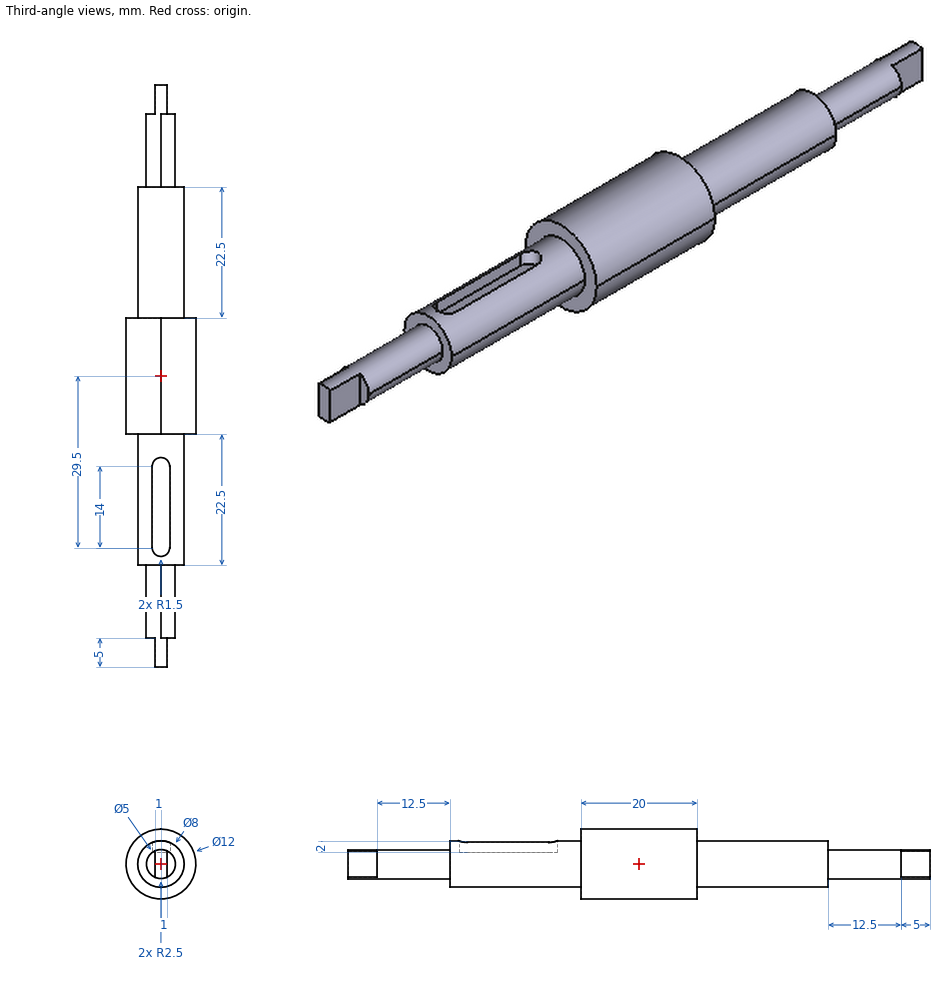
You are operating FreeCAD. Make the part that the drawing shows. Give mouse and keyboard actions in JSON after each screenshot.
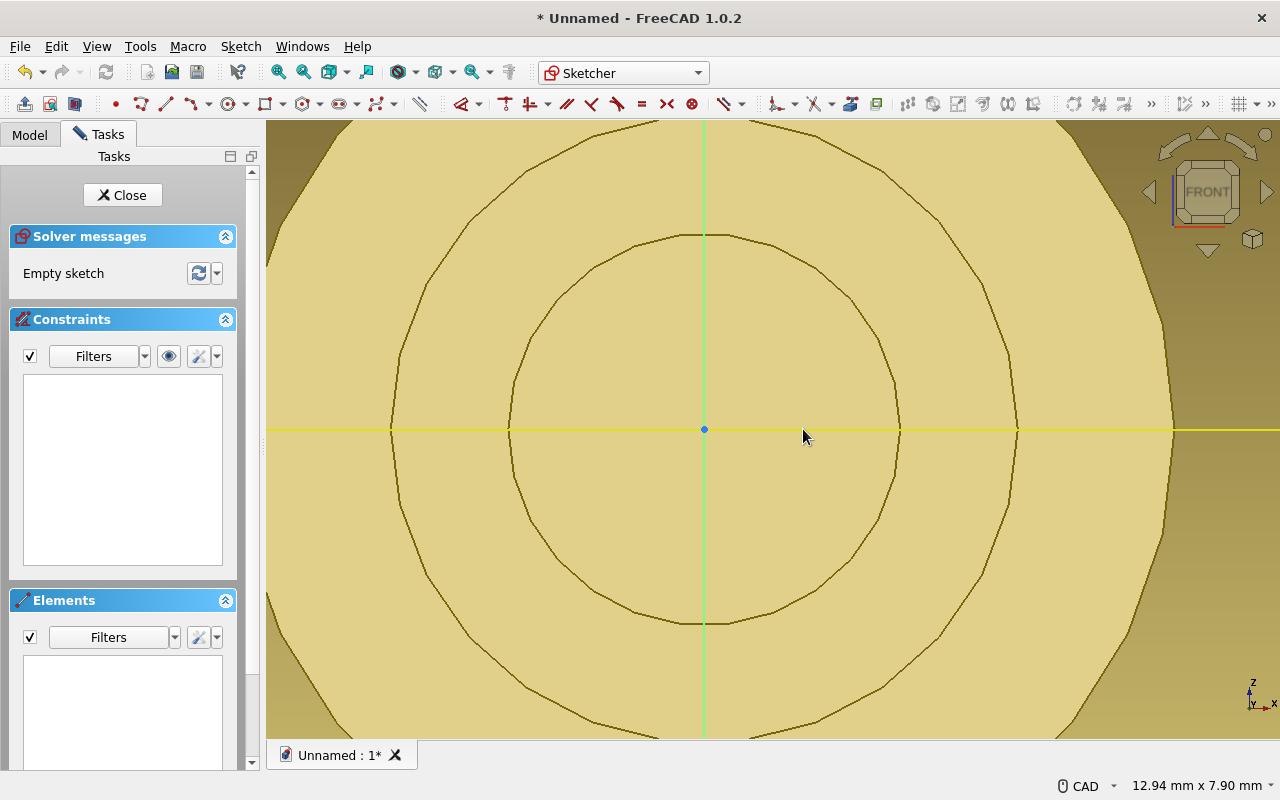
{"action": "left_click", "coordinate": [166, 104]}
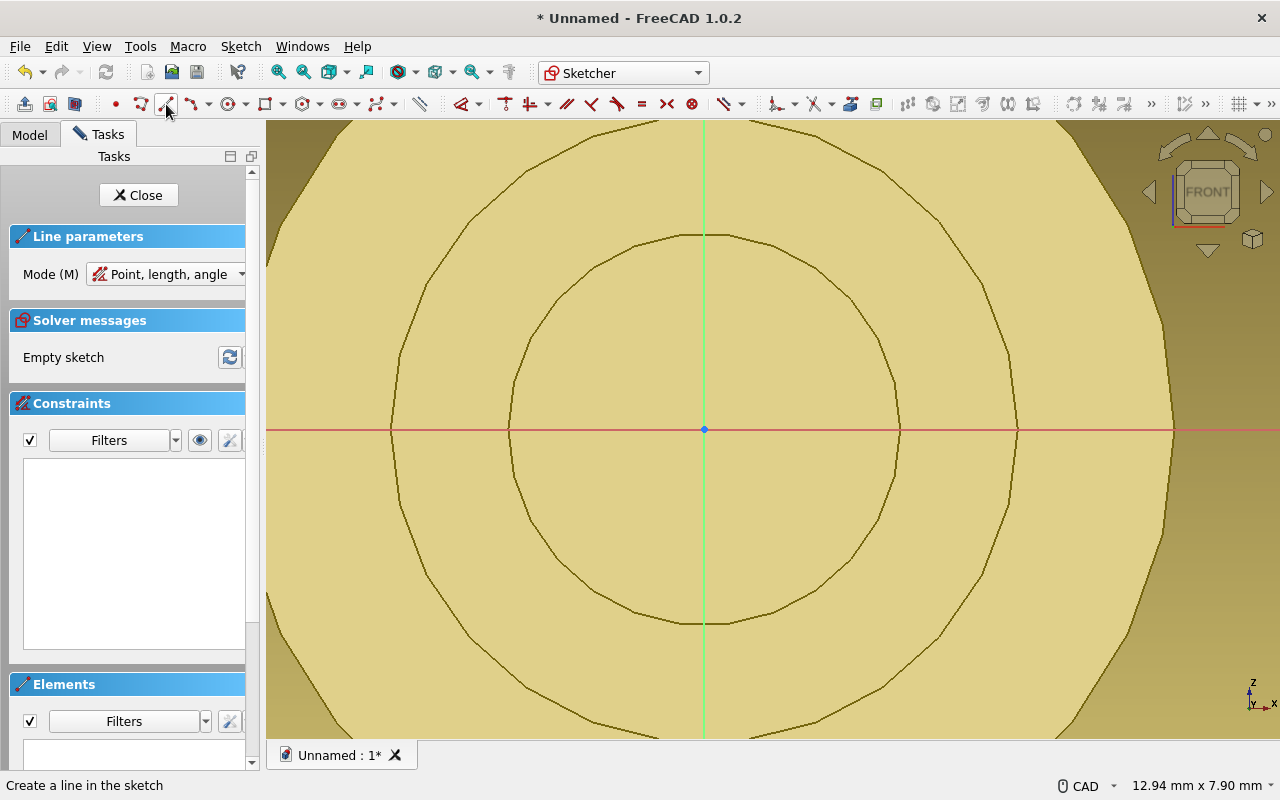
{"action": "left_click", "coordinate": [626, 250]}
{"action": "left_click", "coordinate": [626, 609]}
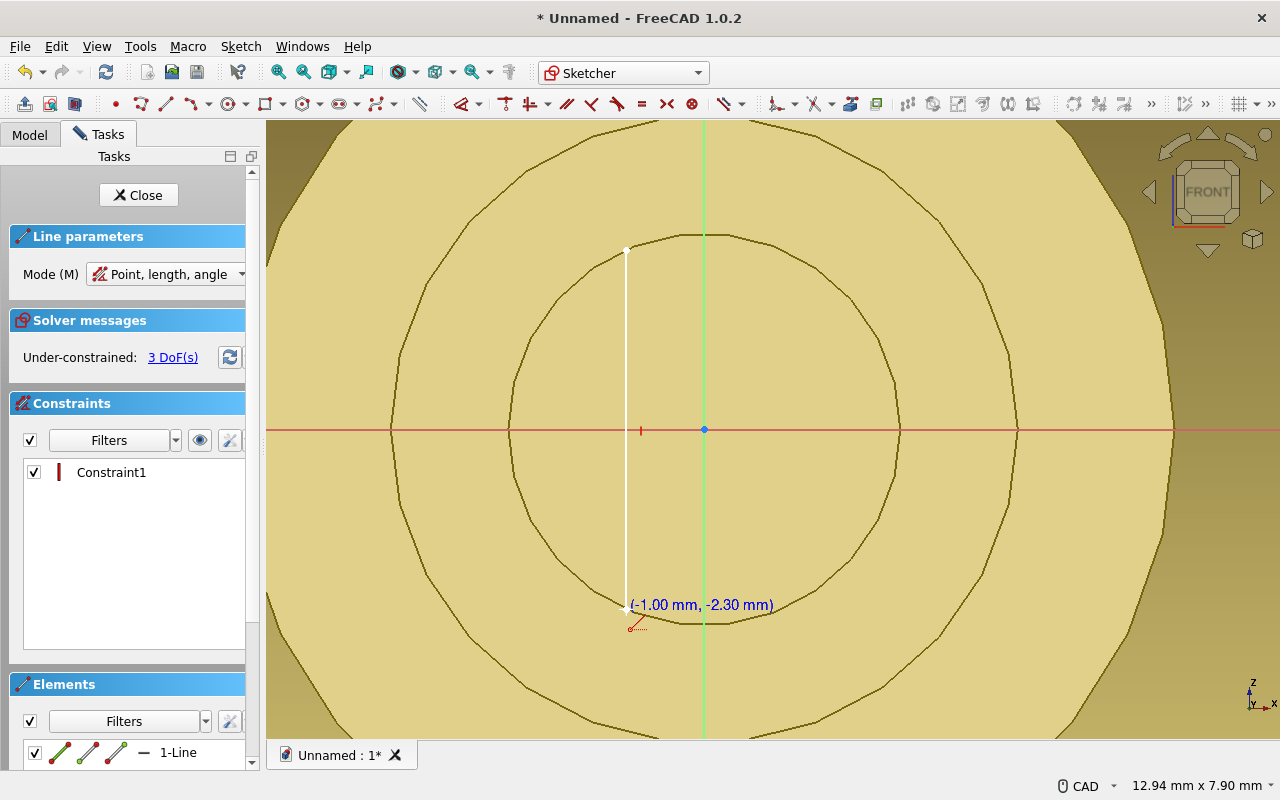
{"action": "left_click", "coordinate": [783, 609]}
{"action": "left_click", "coordinate": [783, 250]}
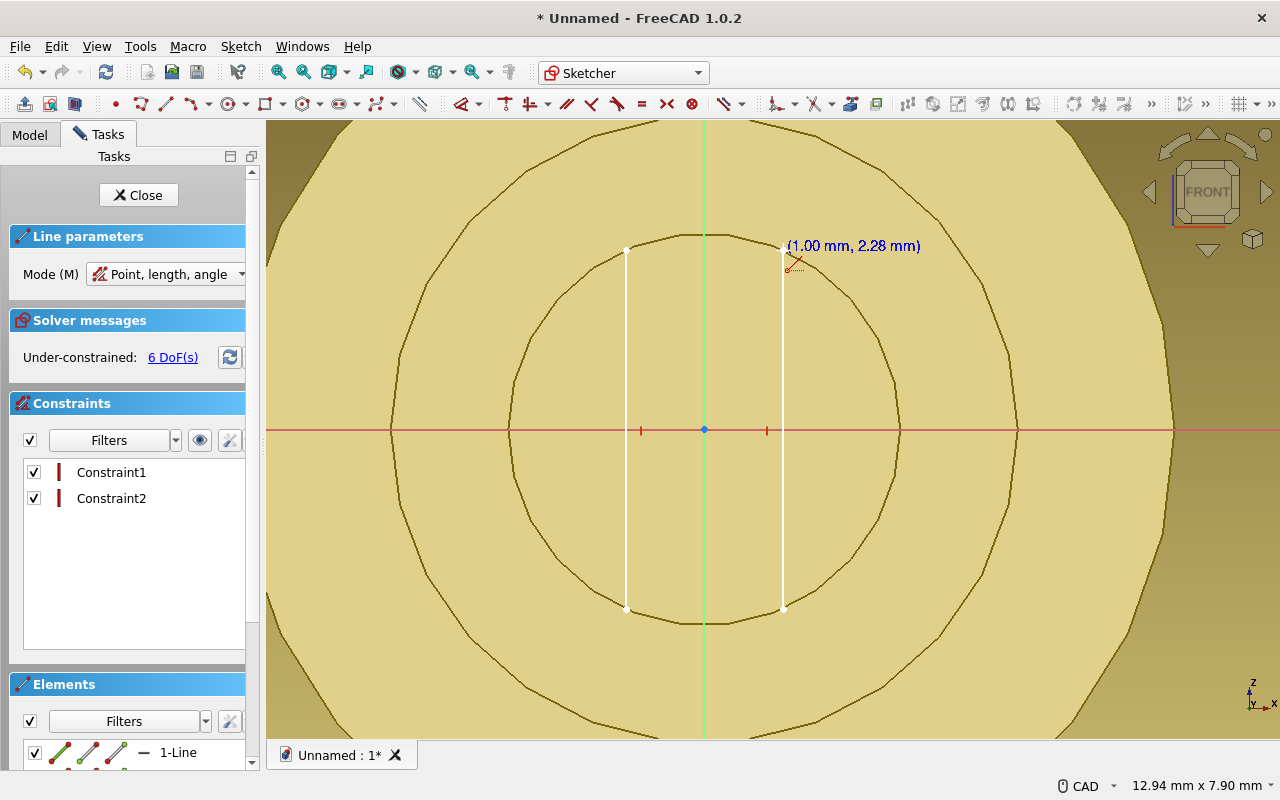
{"action": "left_click", "coordinate": [190, 104]}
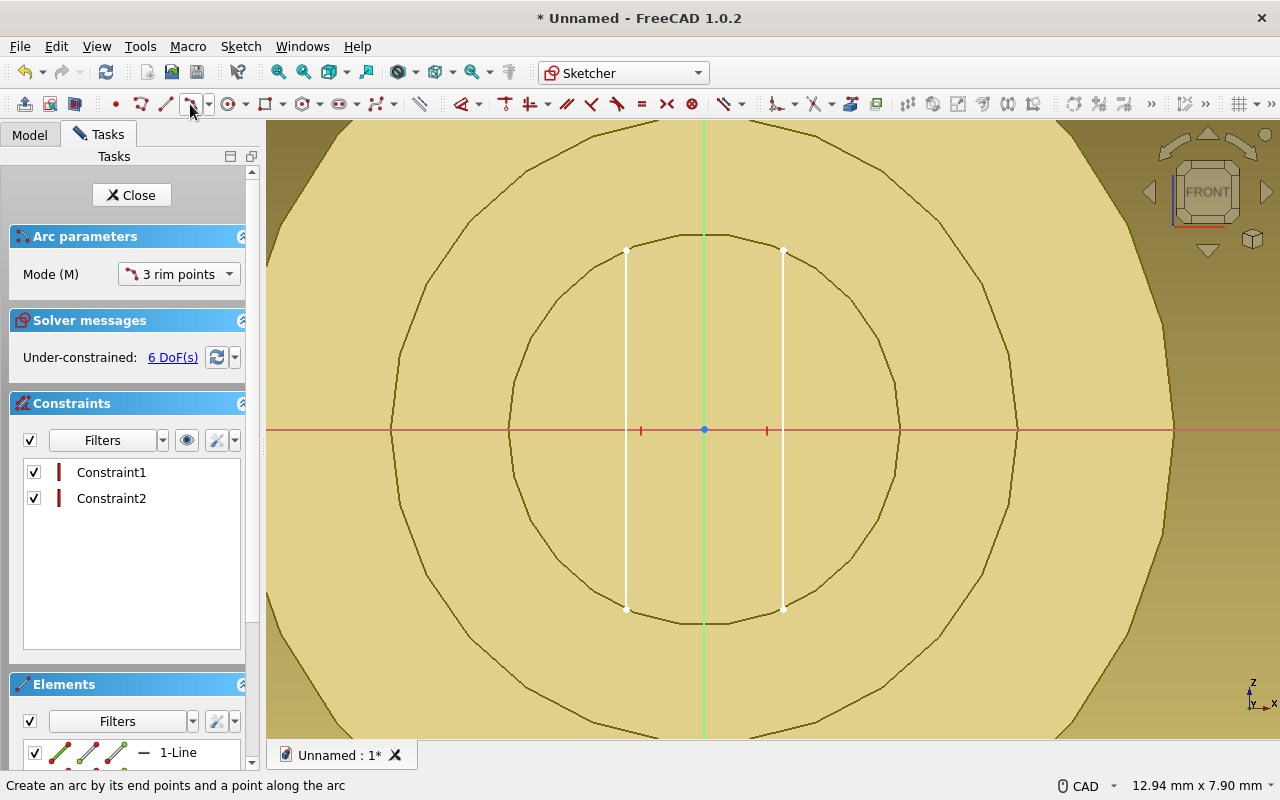
{"action": "left_click", "coordinate": [626, 610]}
{"action": "left_click", "coordinate": [783, 610]}
{"action": "left_click", "coordinate": [688, 625]}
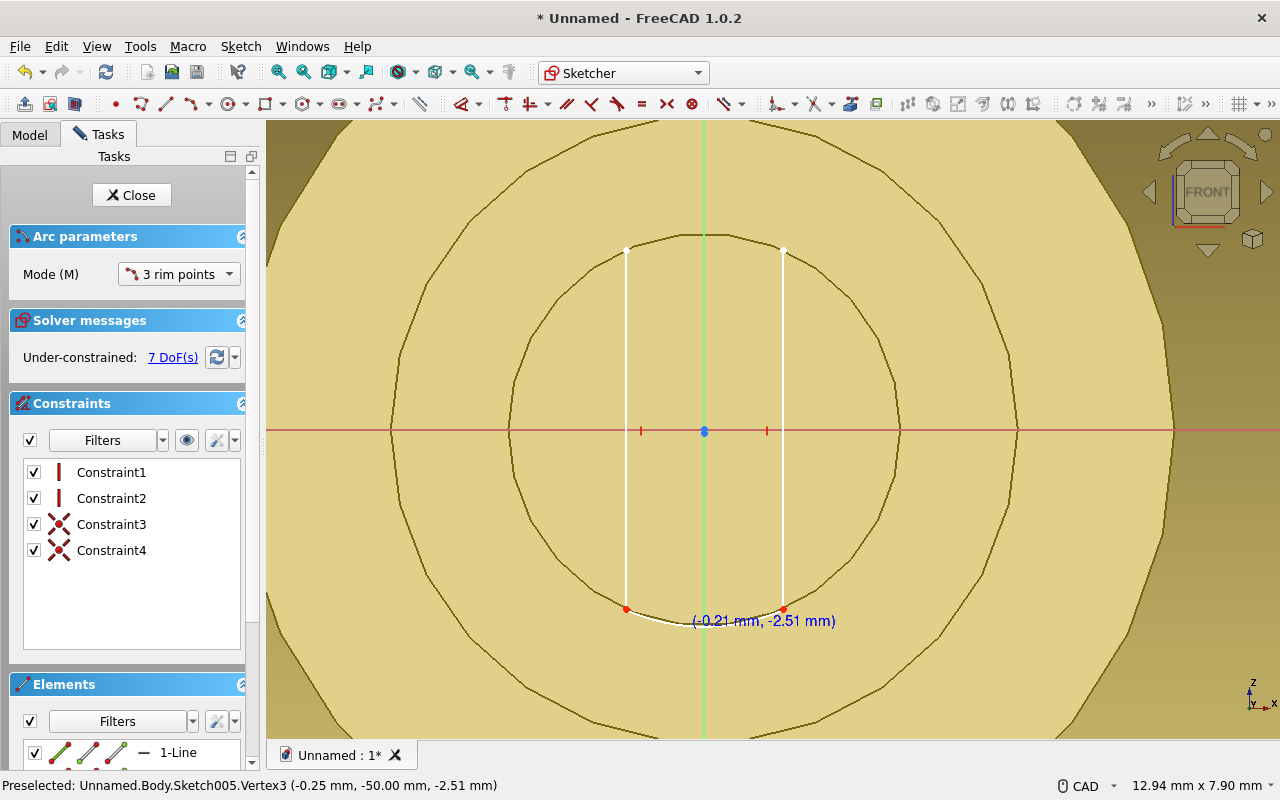
{"action": "left_click", "coordinate": [783, 251]}
{"action": "left_click", "coordinate": [626, 251]}
{"action": "left_click", "coordinate": [720, 234]}
{"action": "key", "text": "Escape"}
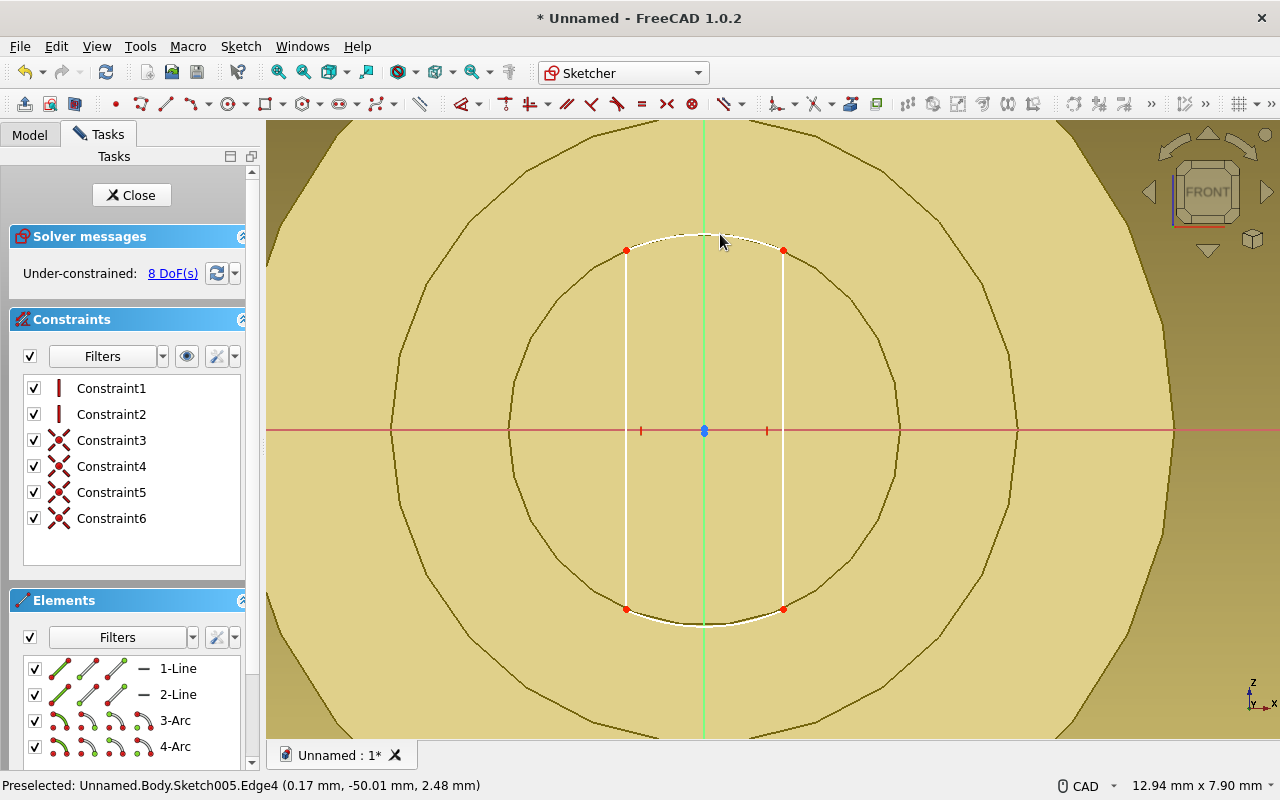
{"action": "left_click", "coordinate": [672, 624]}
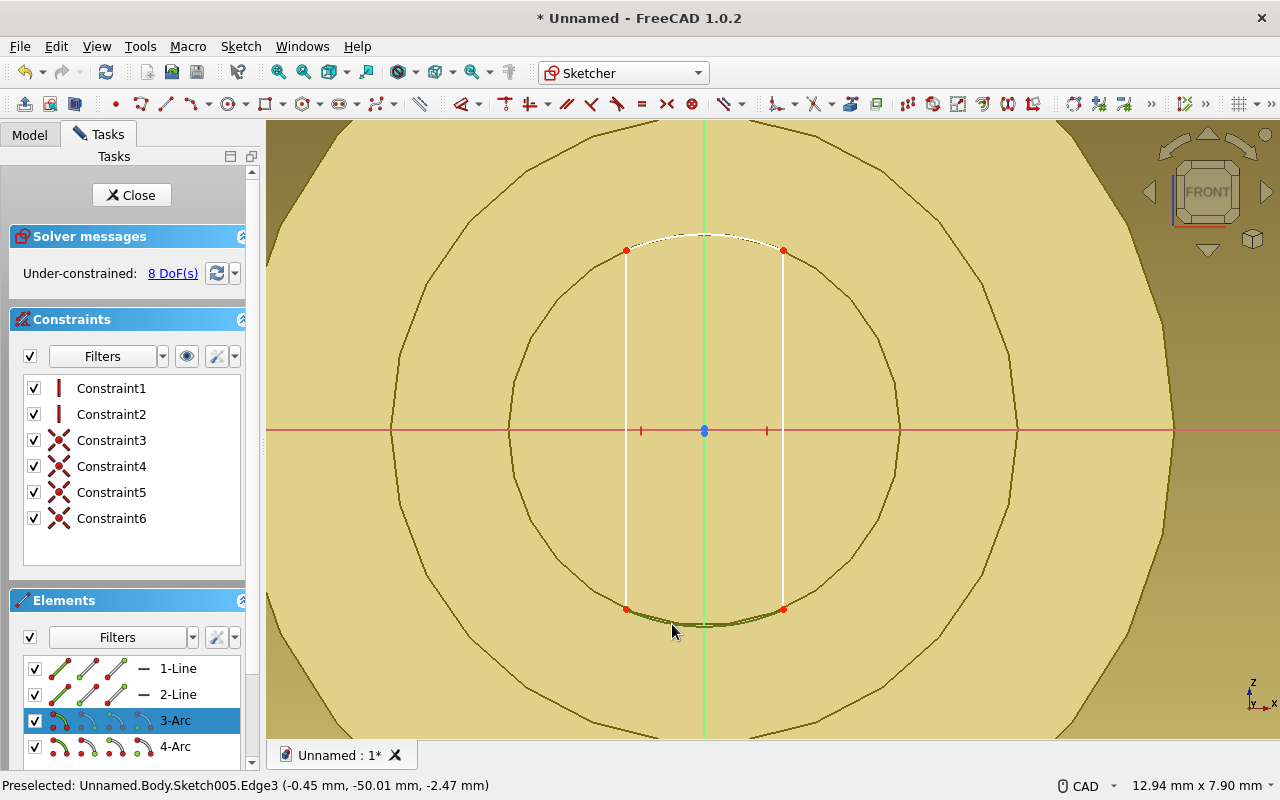
{"action": "left_click", "coordinate": [737, 237]}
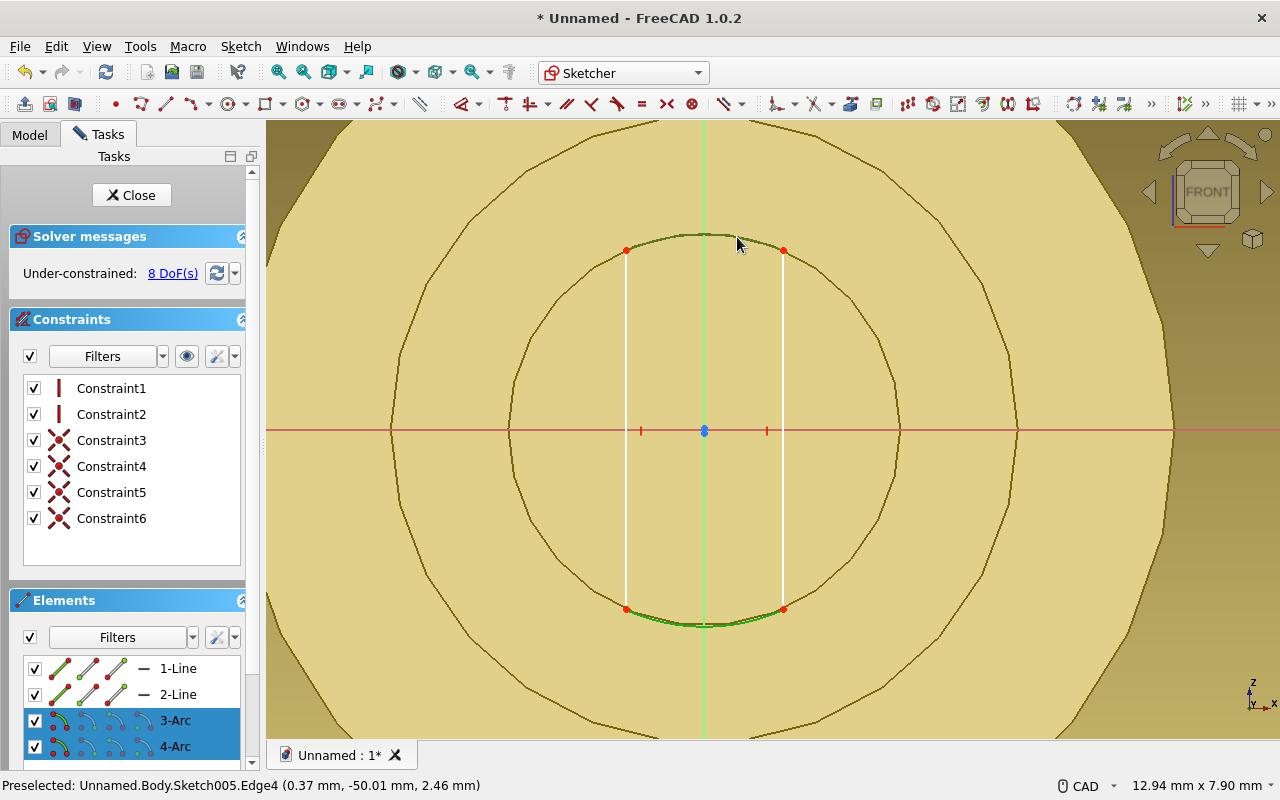
{"action": "key", "text": "c"}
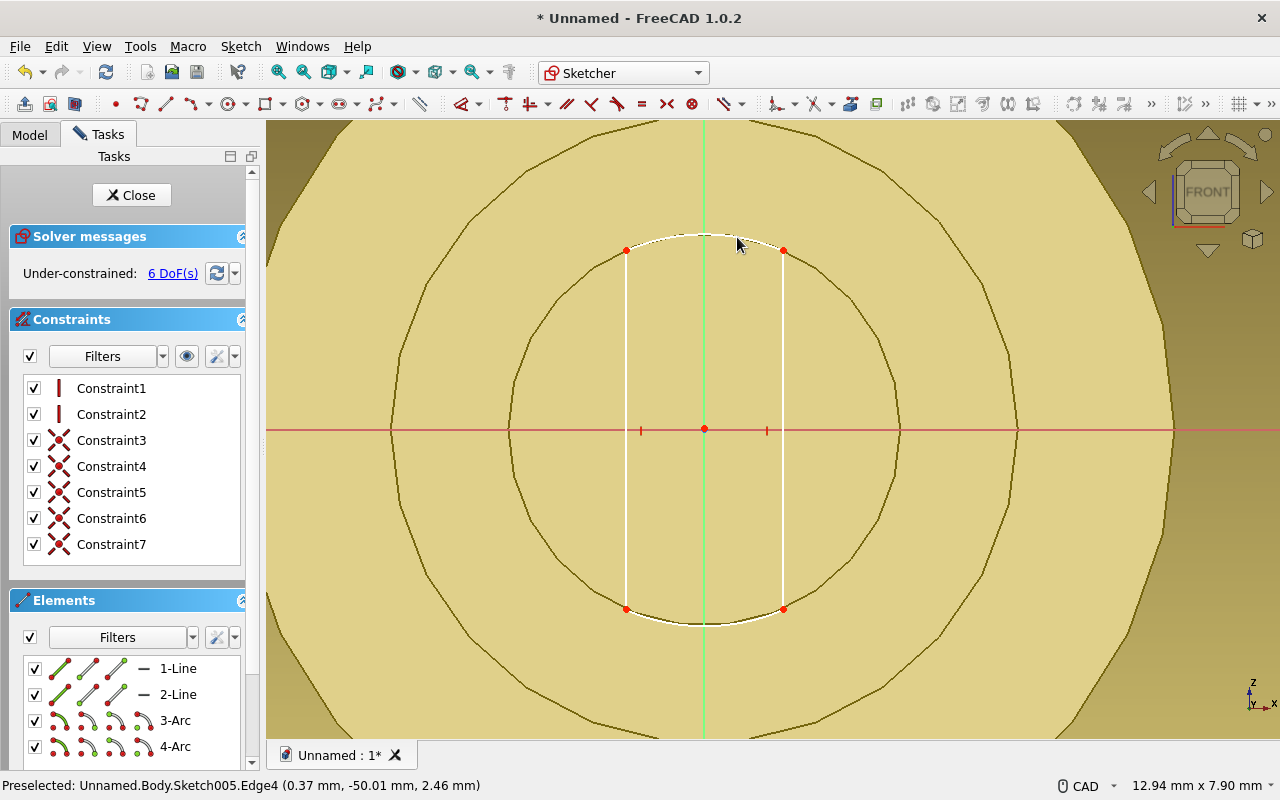
{"action": "left_click_drag", "start_coordinate": [694, 418], "coordinate": [714, 439]}